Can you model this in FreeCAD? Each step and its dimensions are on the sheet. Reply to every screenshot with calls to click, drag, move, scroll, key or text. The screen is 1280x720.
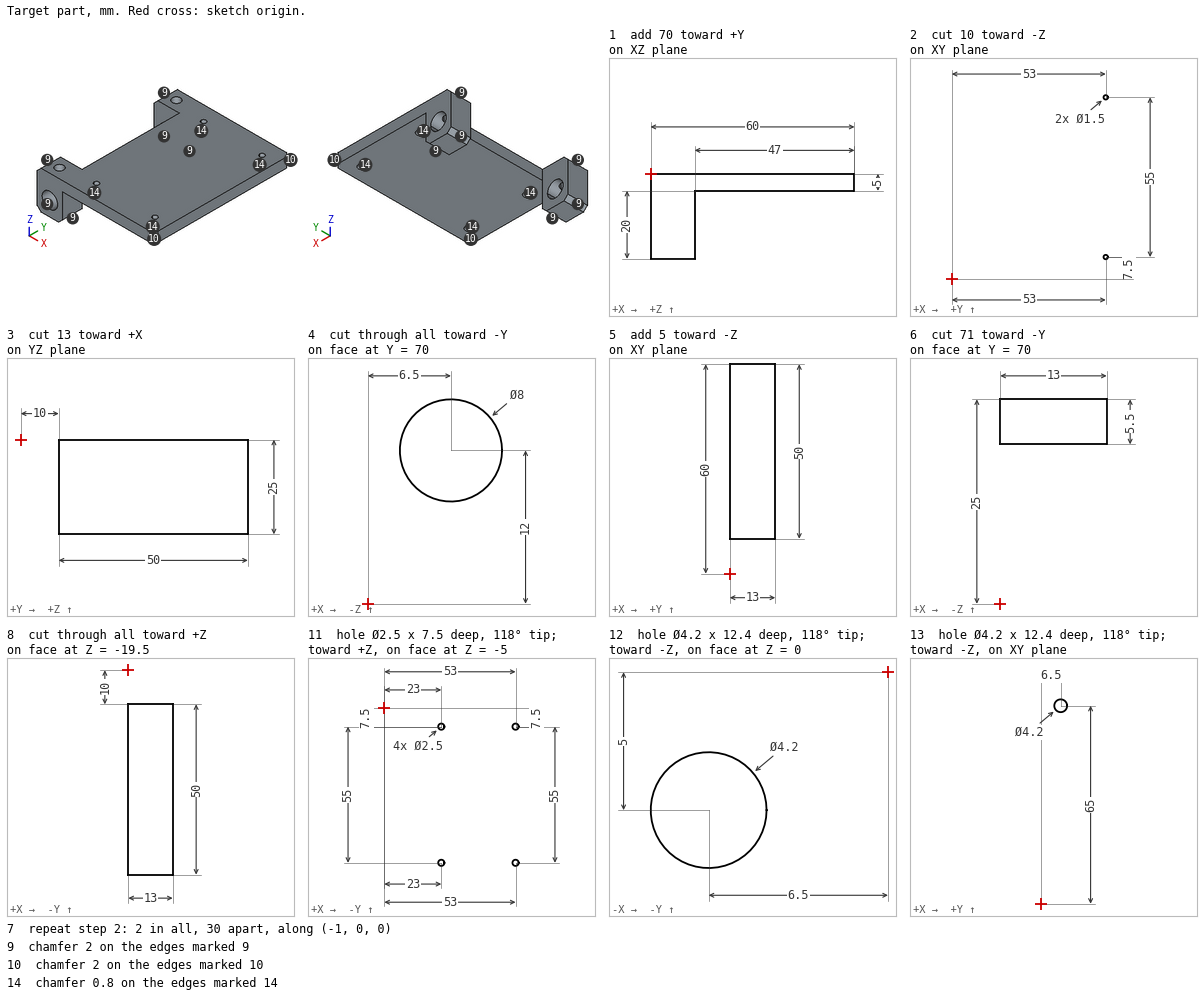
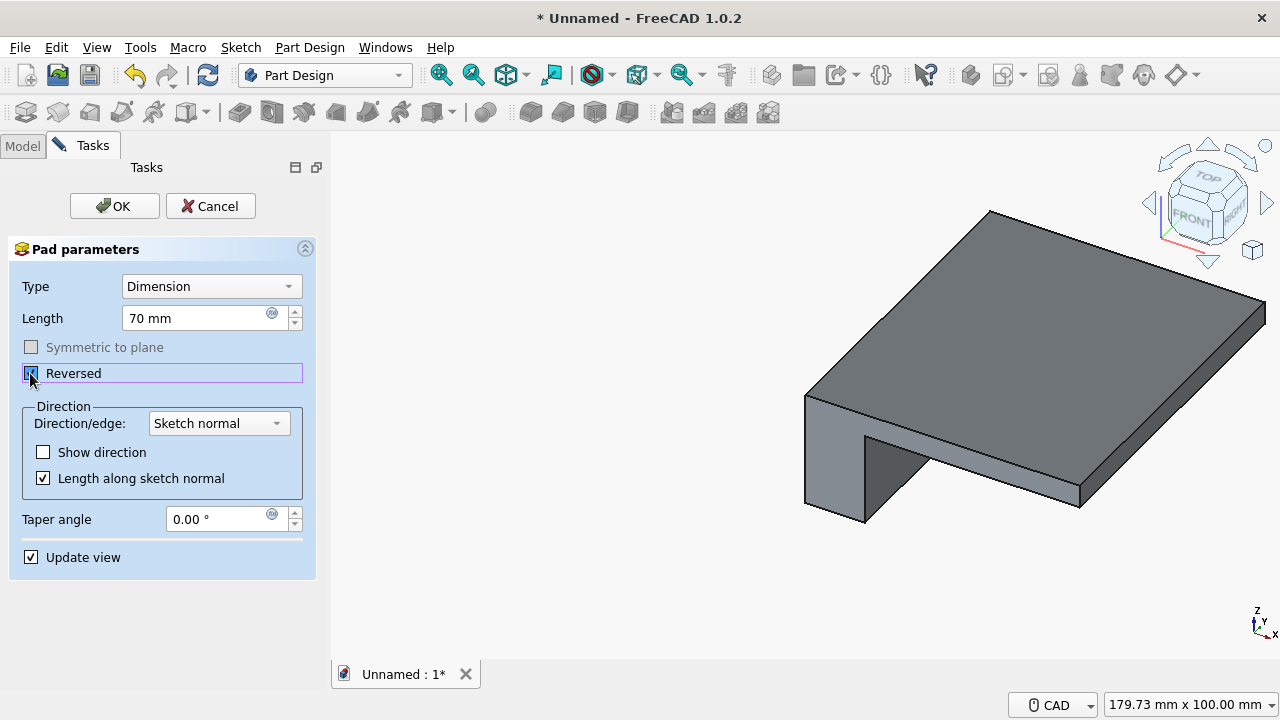
click(115, 206)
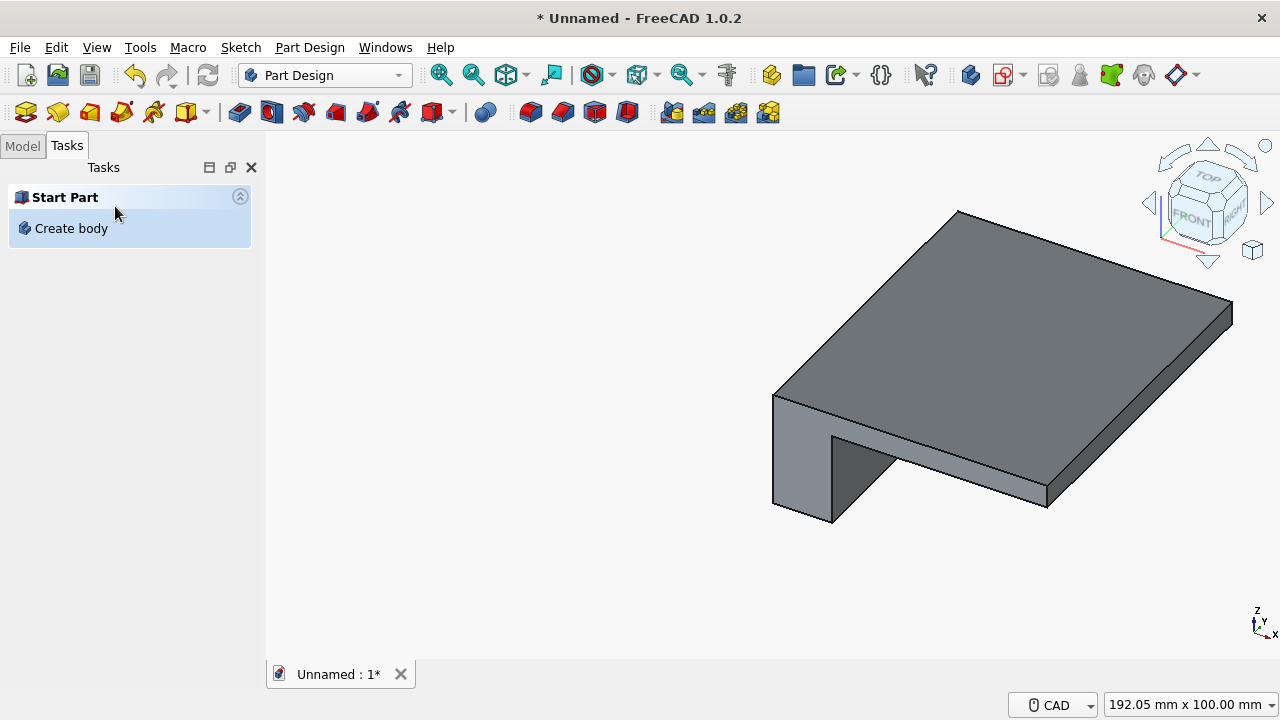
click(1004, 76)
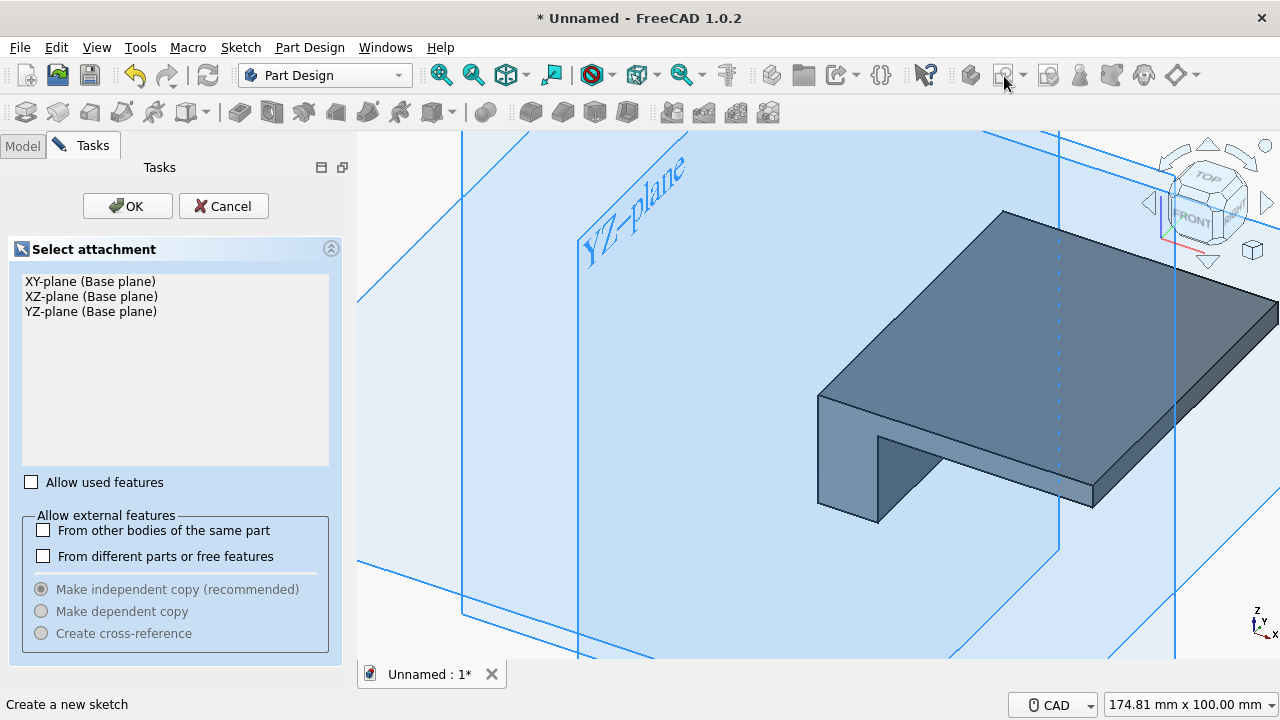
click(82, 282)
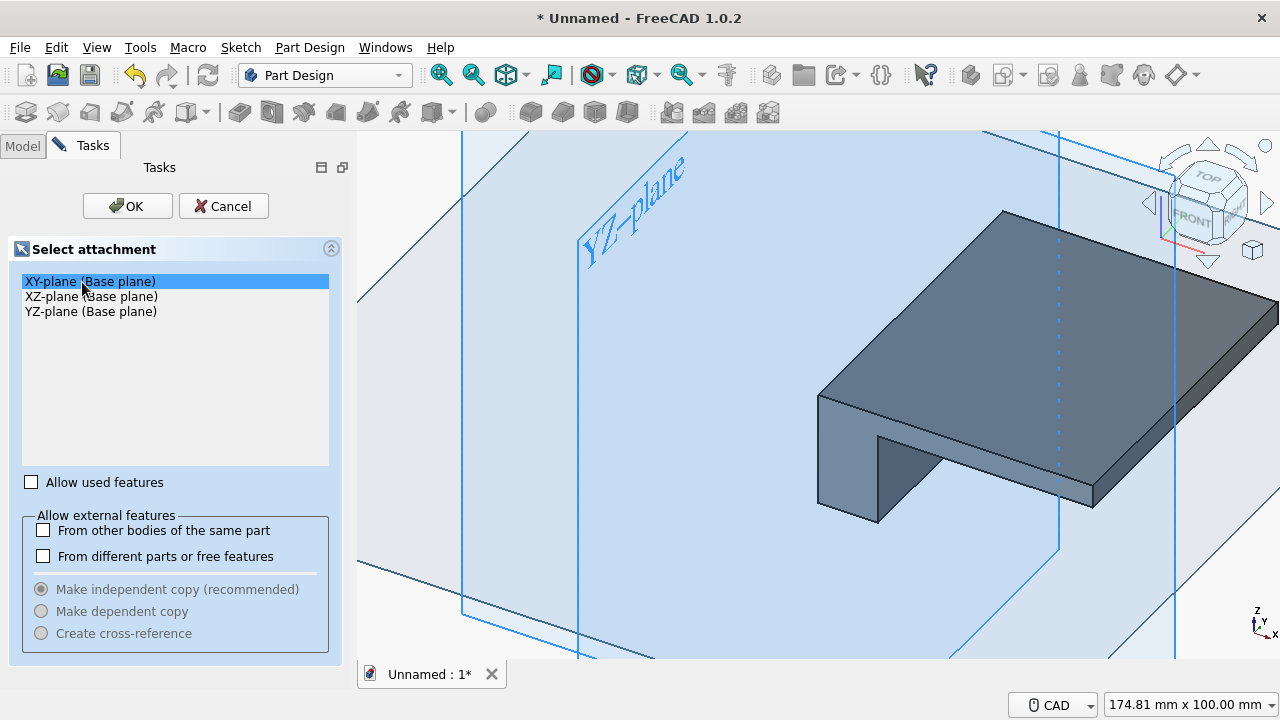
click(128, 206)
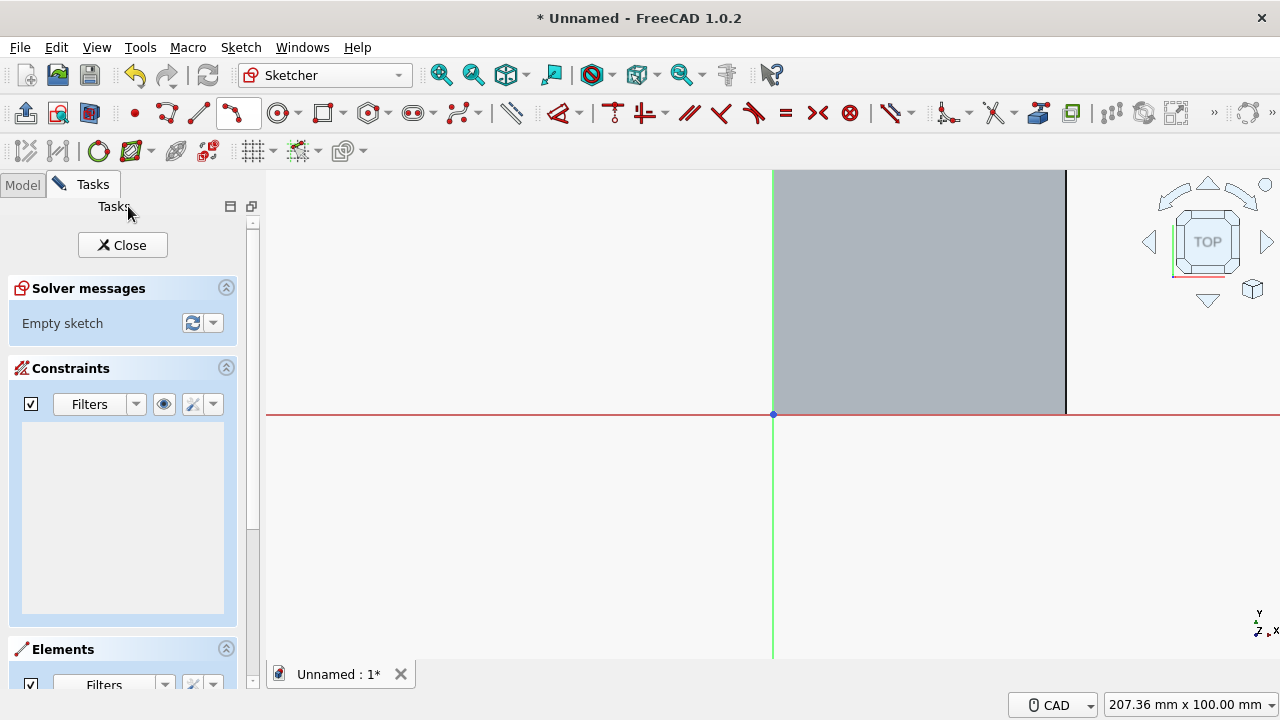
scroll(298, 631, down, 2)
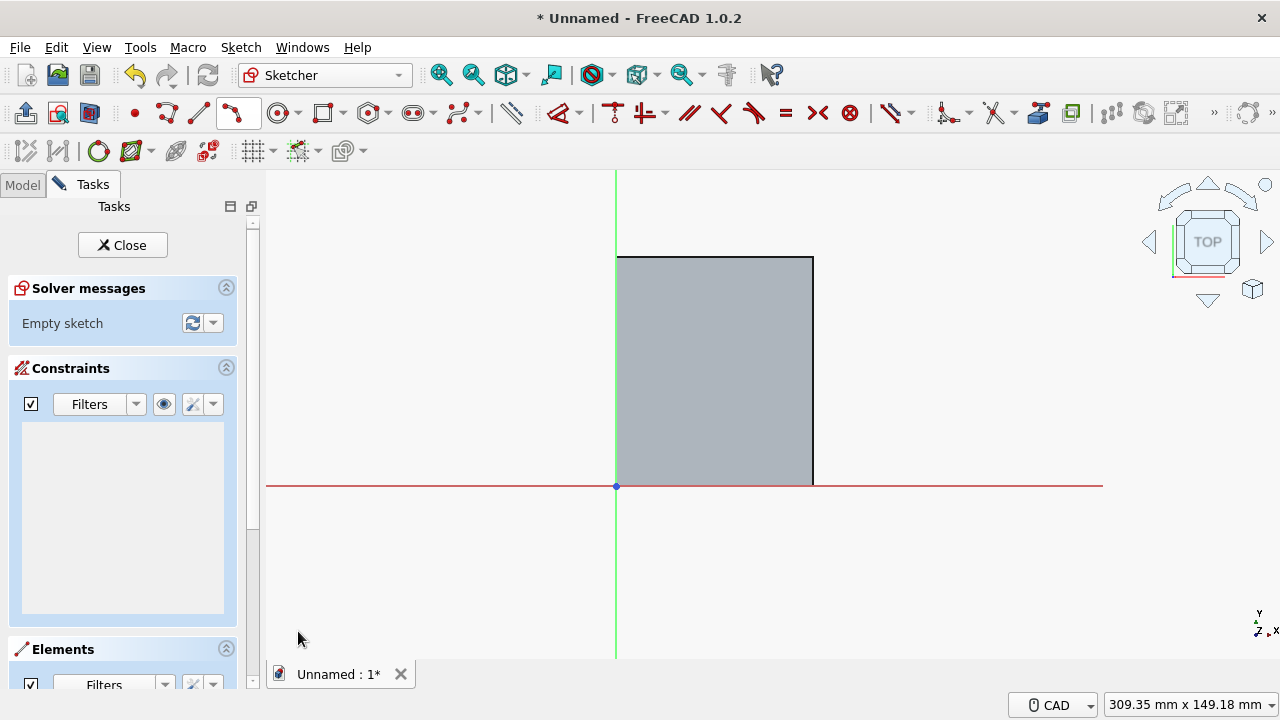
scroll(705, 318, up, 2)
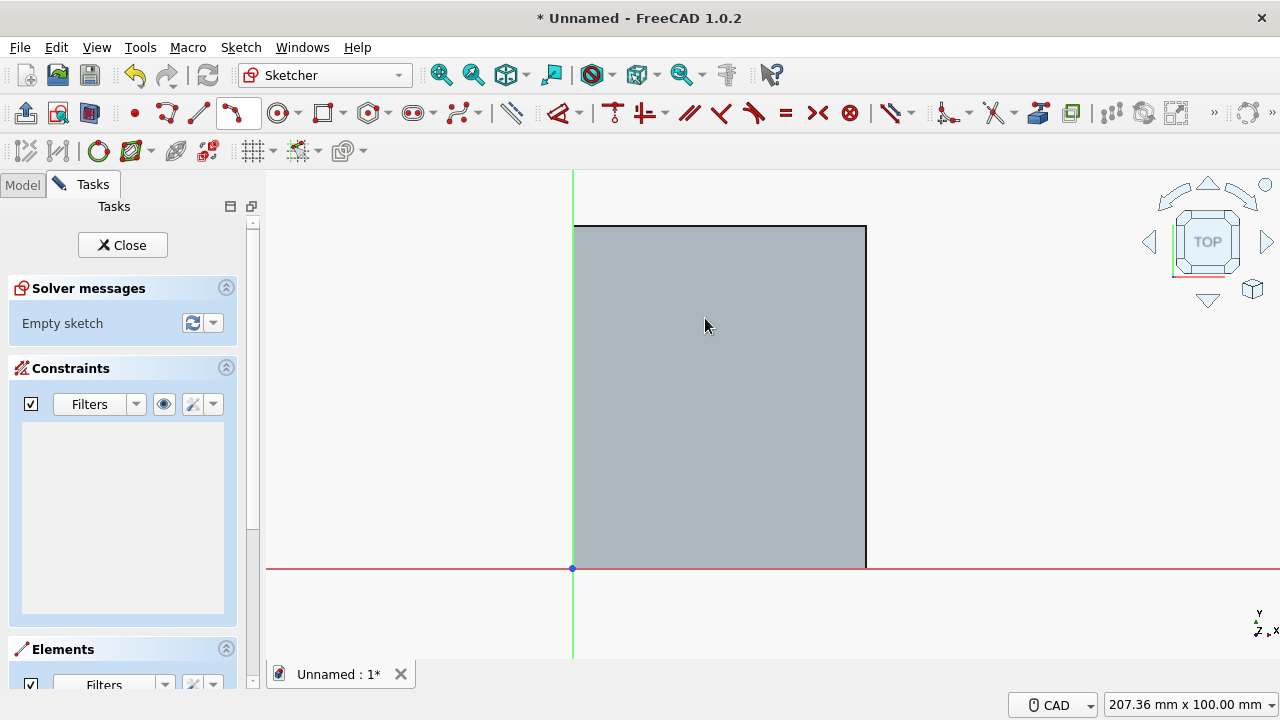
click(278, 114)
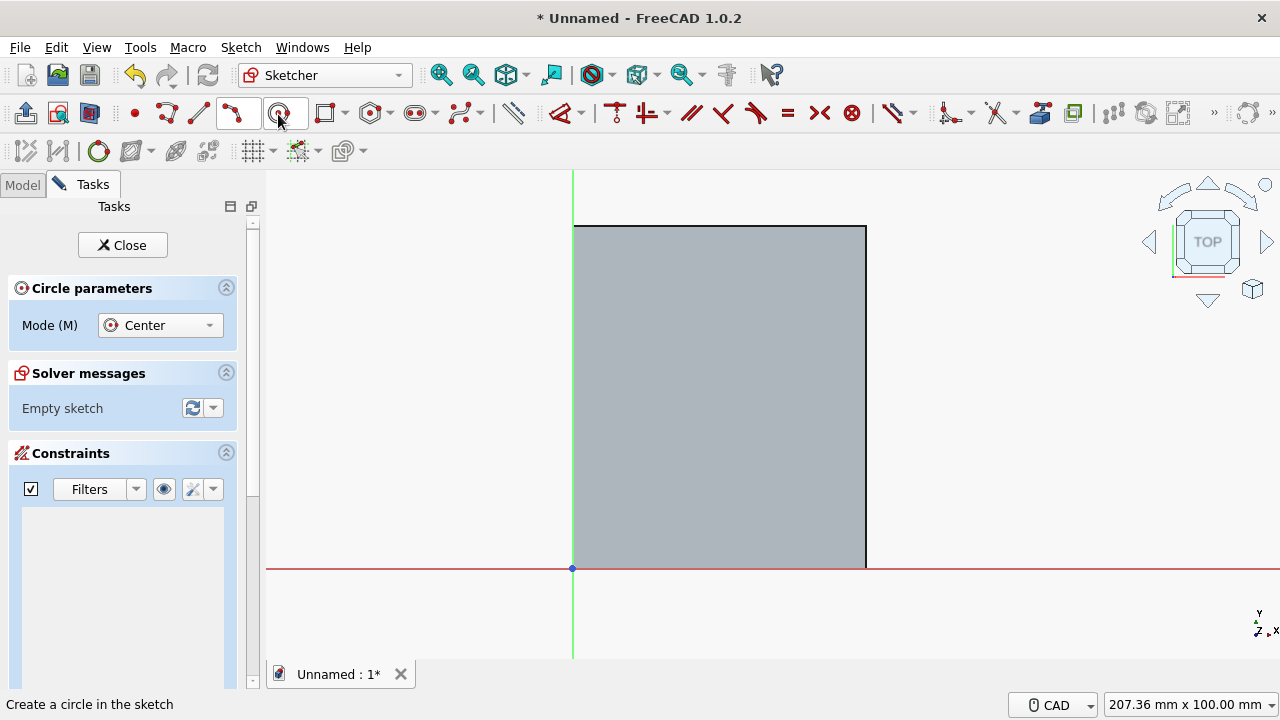
scroll(832, 263, up, 10)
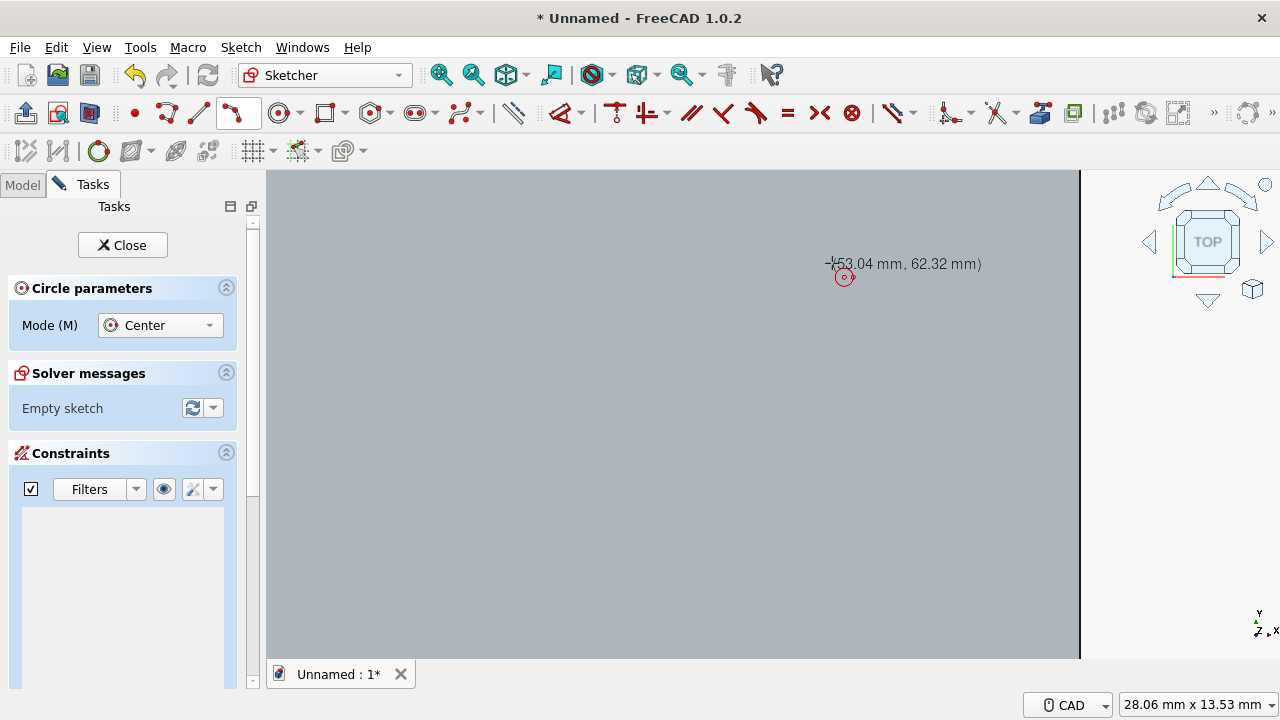
scroll(833, 264, down, 10)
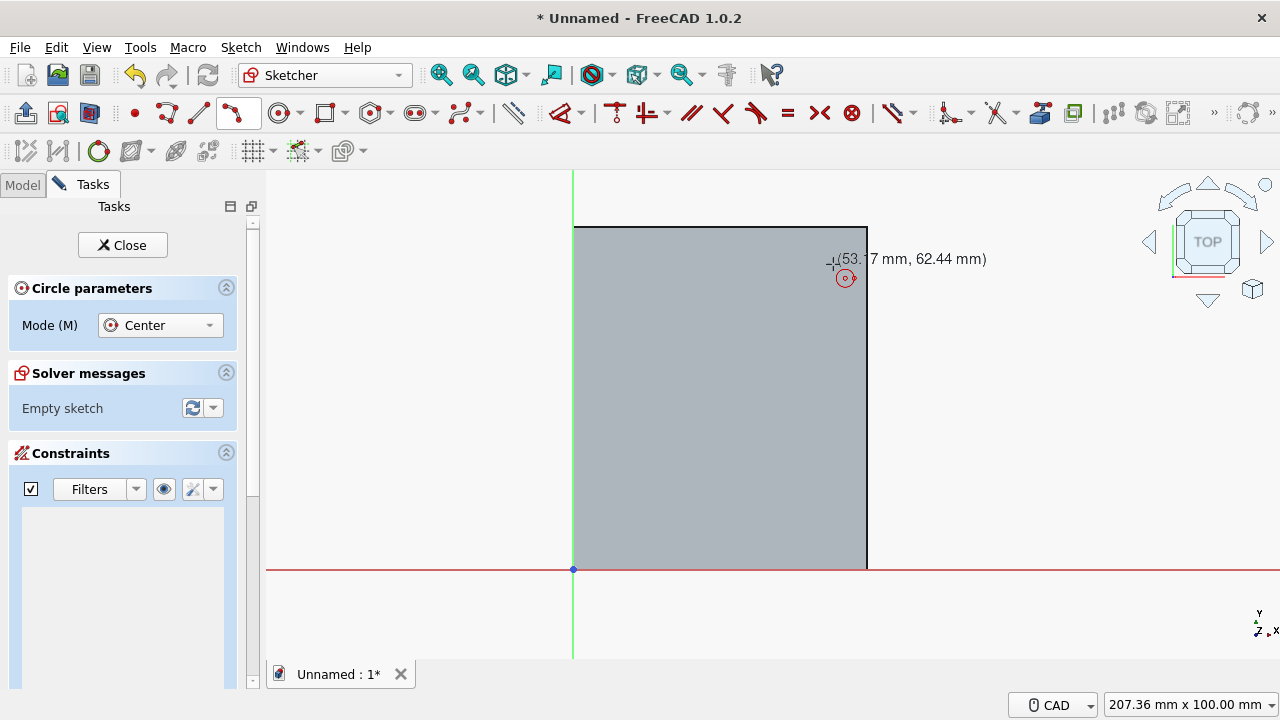
click(833, 264)
move(835, 261)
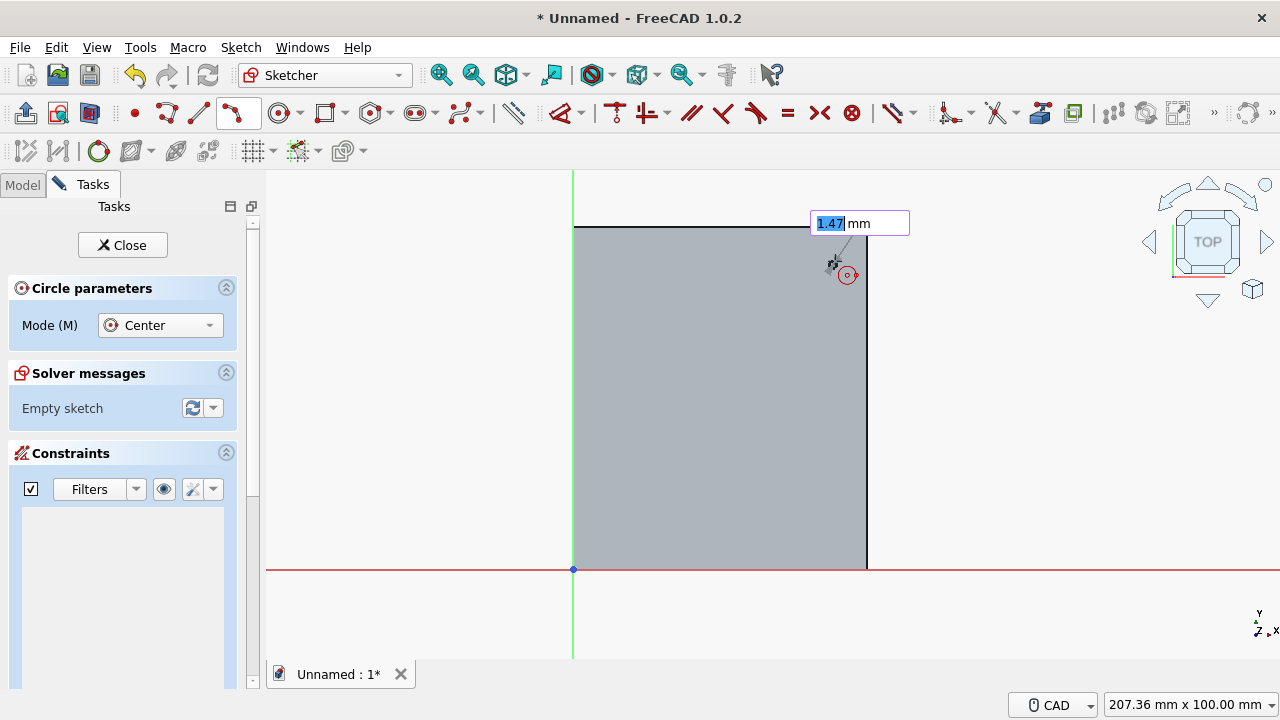
text(1.5)
key(Return)